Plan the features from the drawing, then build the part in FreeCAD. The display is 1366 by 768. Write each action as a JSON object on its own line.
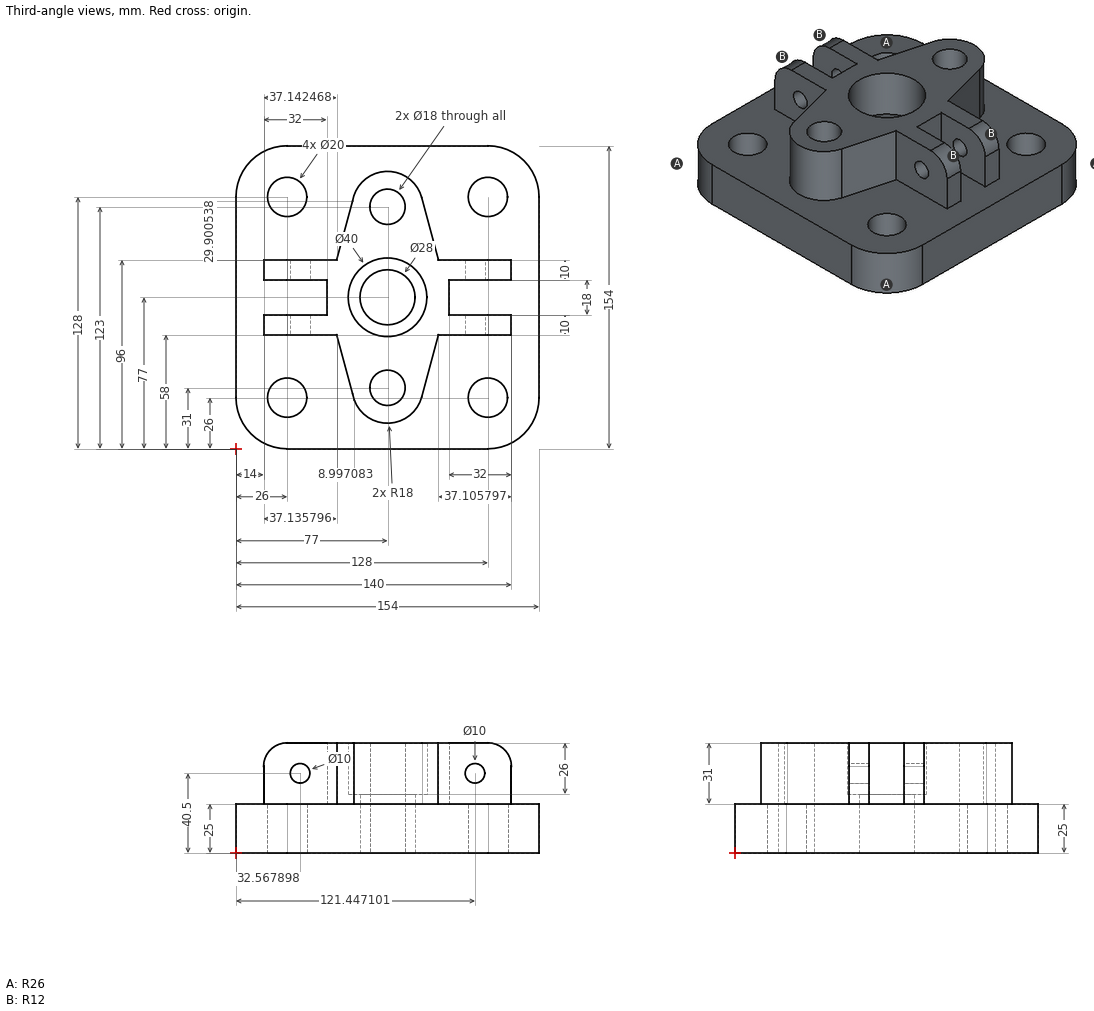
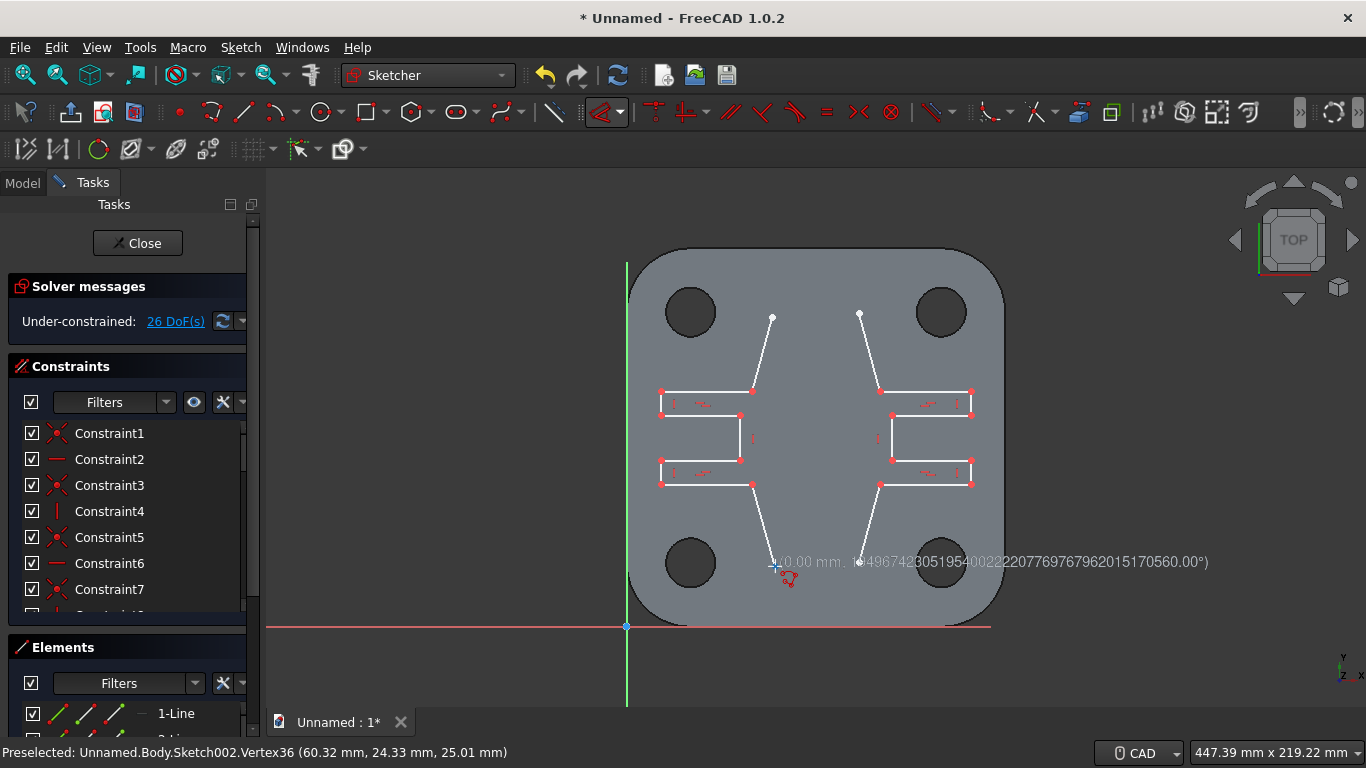
{"action": "key", "text": "g 3 a"}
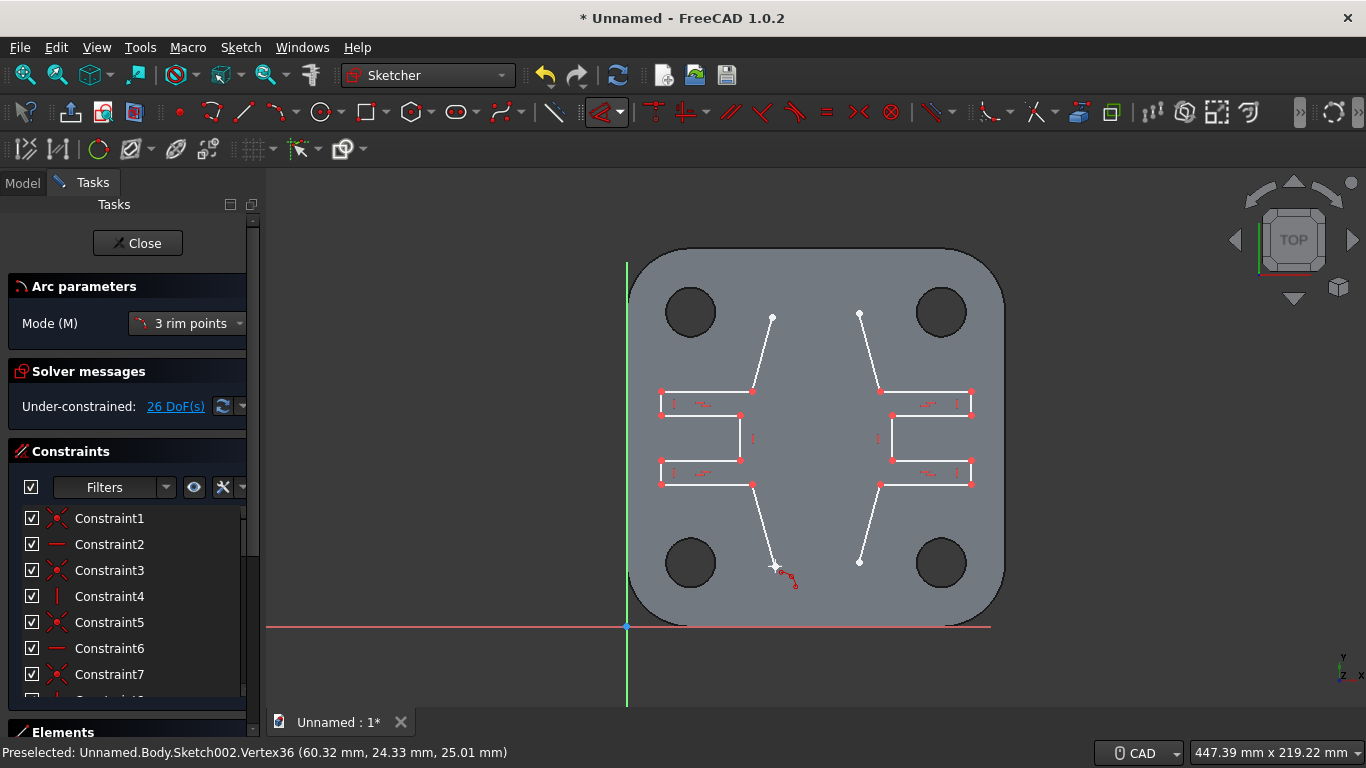
{"action": "left_click", "coordinate": [859, 314]}
{"action": "left_click", "coordinate": [772, 318]}
{"action": "left_click", "coordinate": [814, 280]}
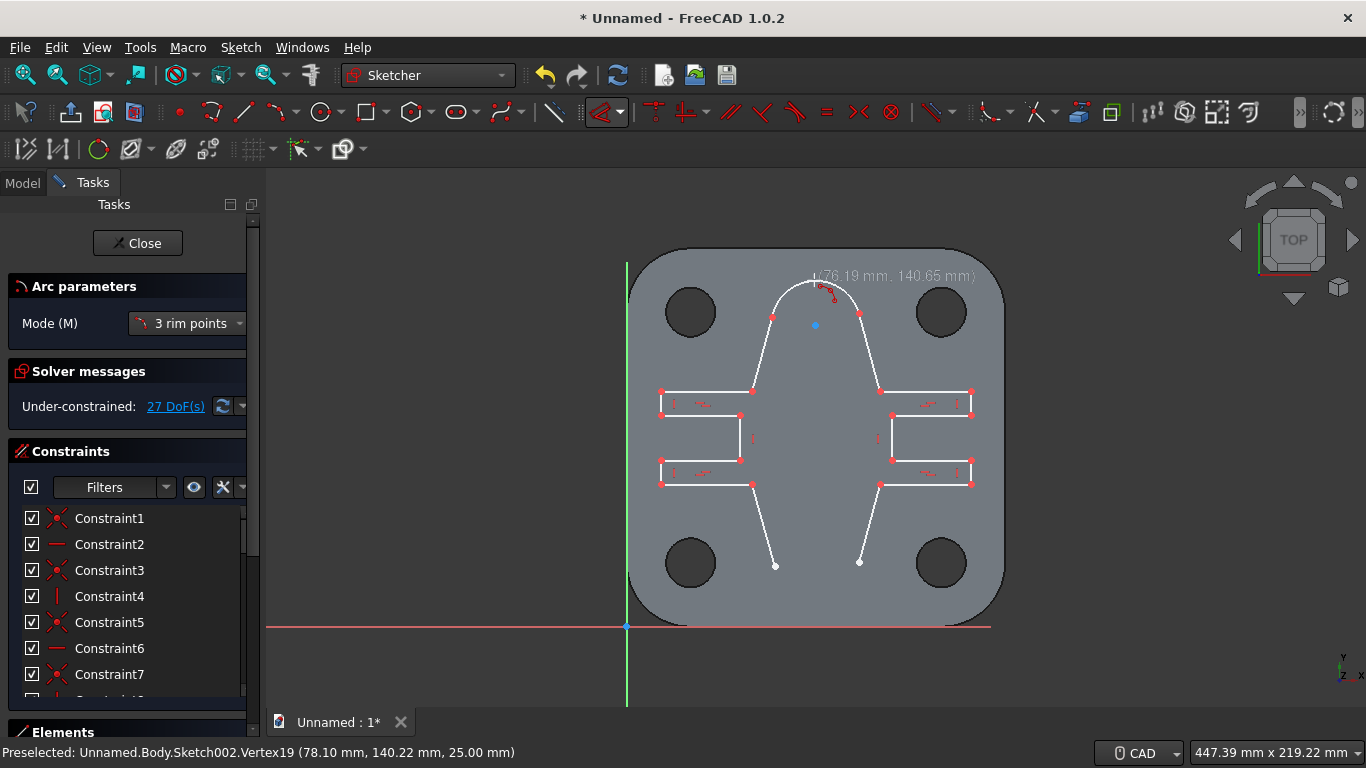
{"action": "left_click", "coordinate": [775, 567]}
{"action": "left_click", "coordinate": [859, 563]}
{"action": "left_click", "coordinate": [818, 595]}
{"action": "key", "text": "Escape"}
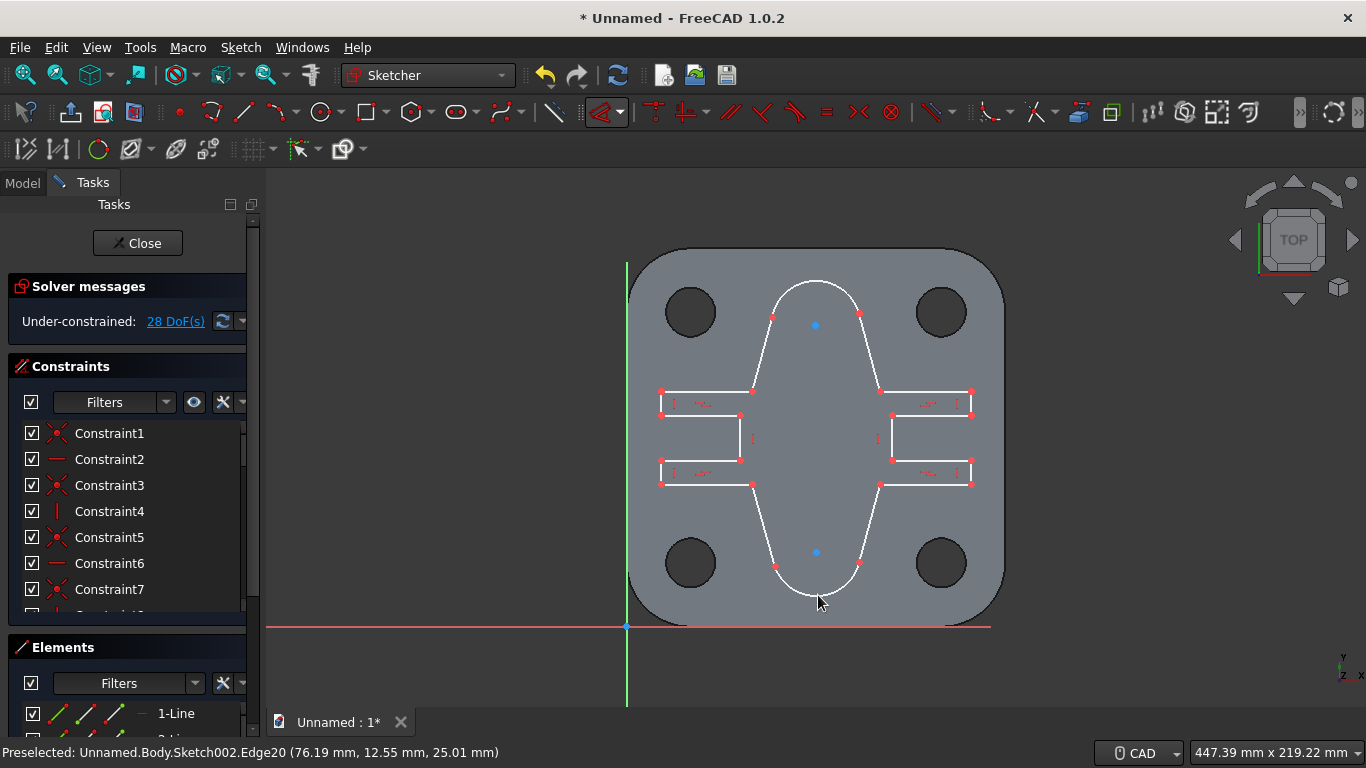
{"action": "left_click", "coordinate": [865, 540]}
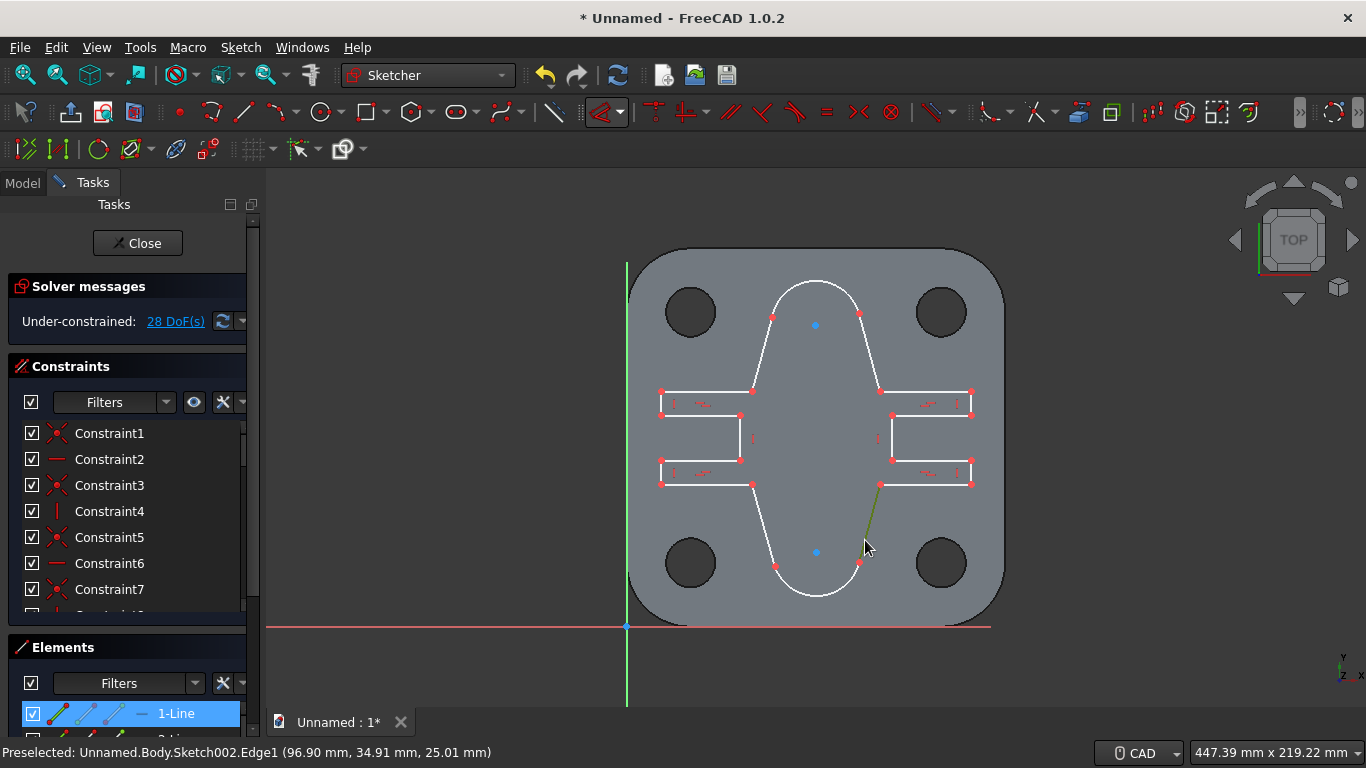
{"action": "left_click", "coordinate": [797, 591]}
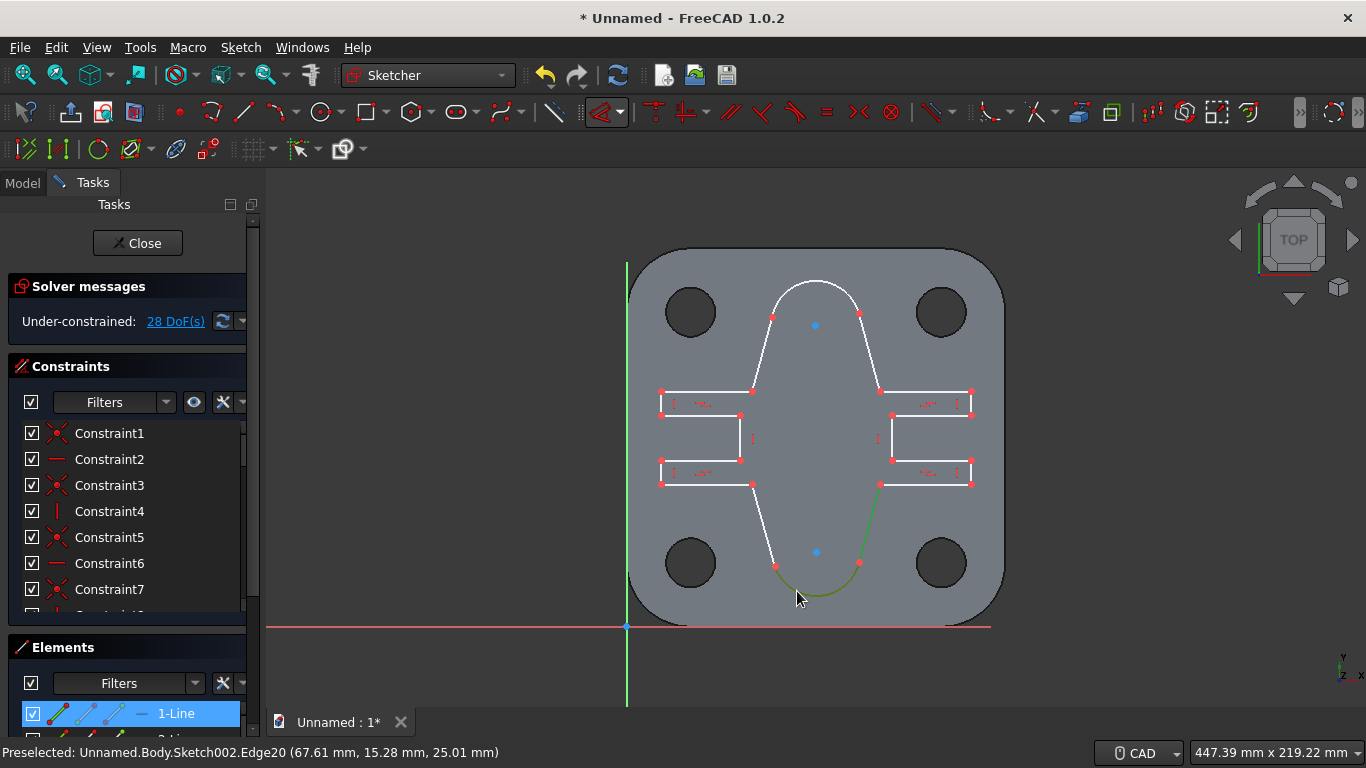
{"action": "left_click", "coordinate": [796, 112]}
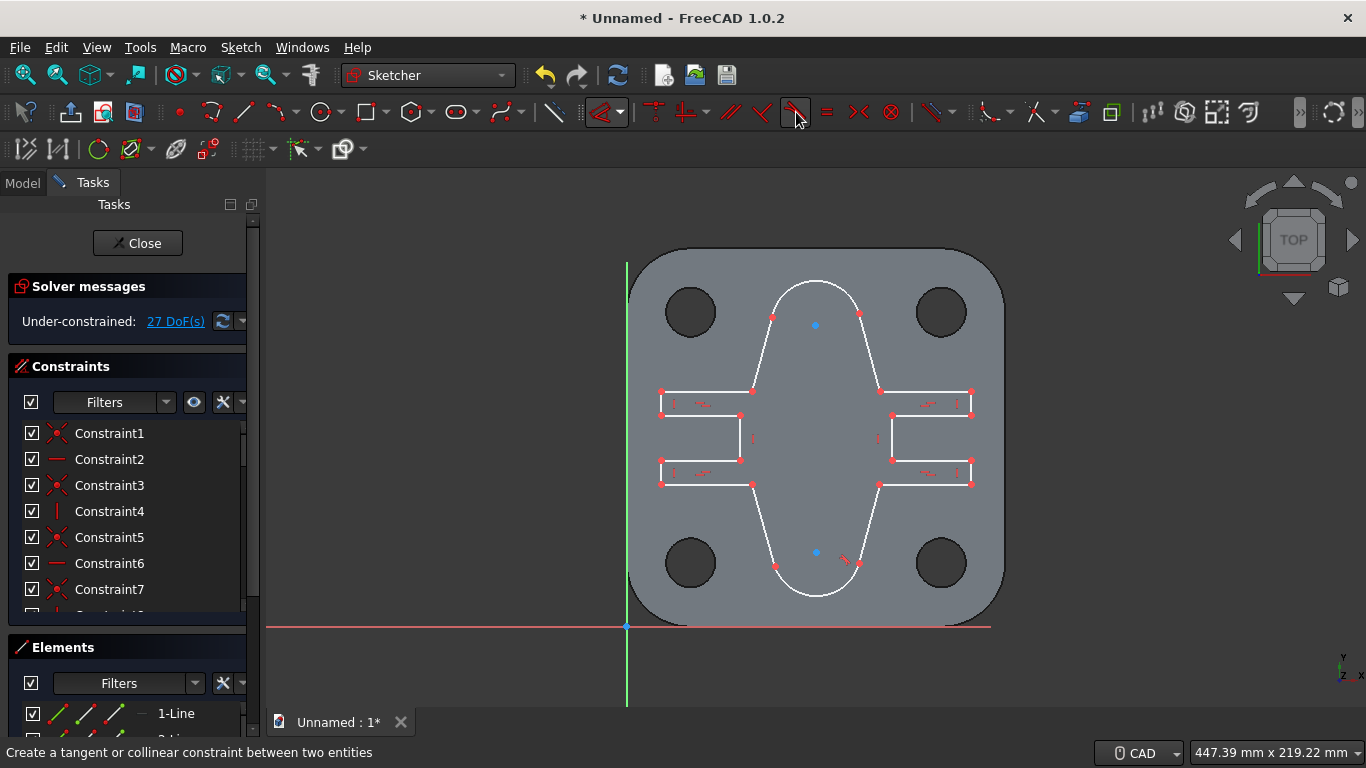
{"action": "left_click", "coordinate": [874, 369]}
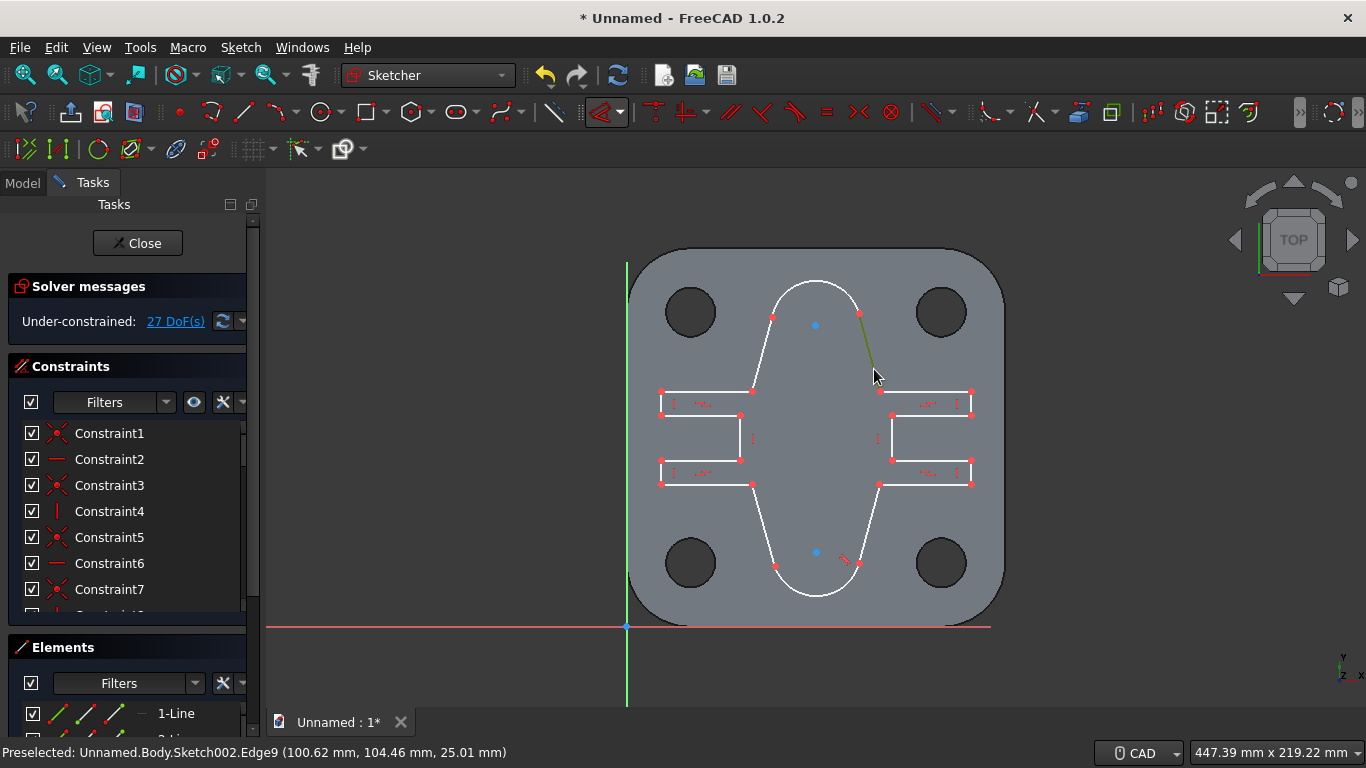
{"action": "left_click", "coordinate": [837, 286]}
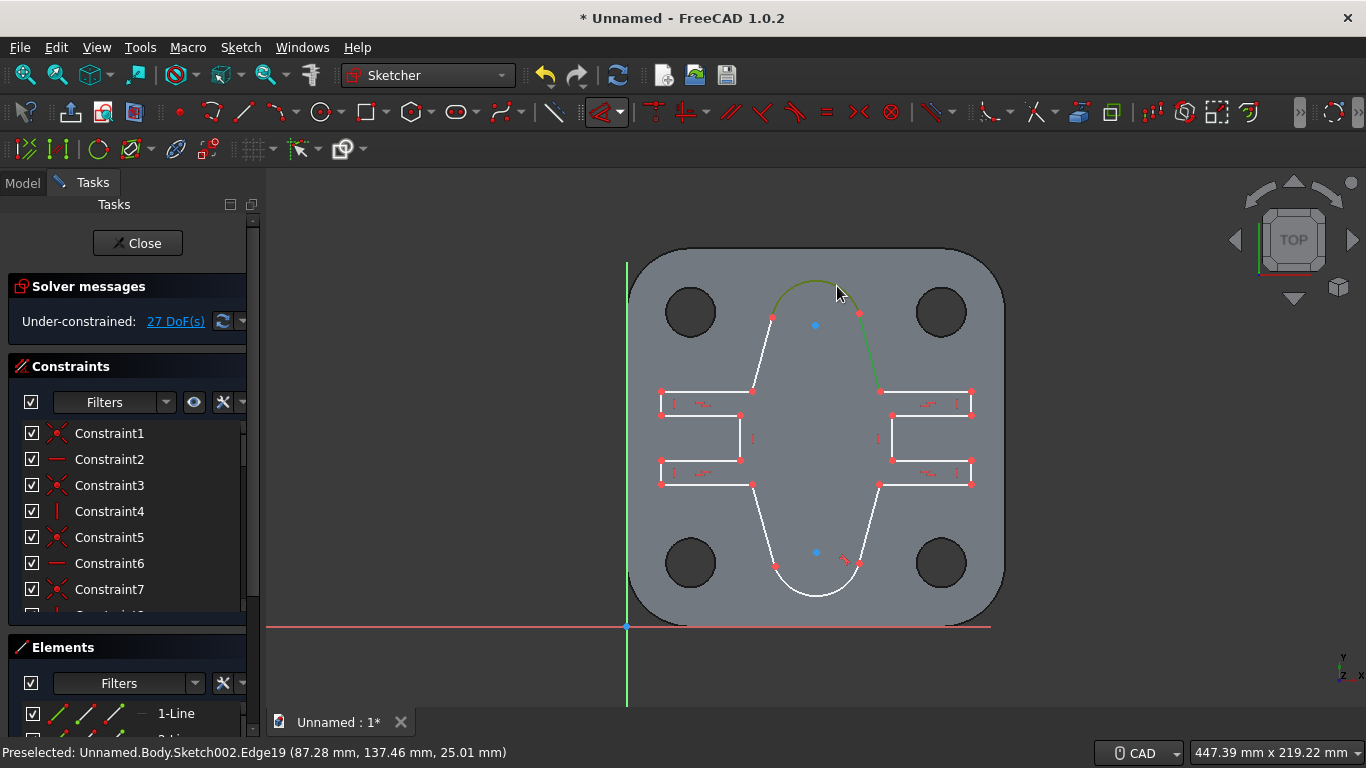
{"action": "left_click", "coordinate": [796, 112]}